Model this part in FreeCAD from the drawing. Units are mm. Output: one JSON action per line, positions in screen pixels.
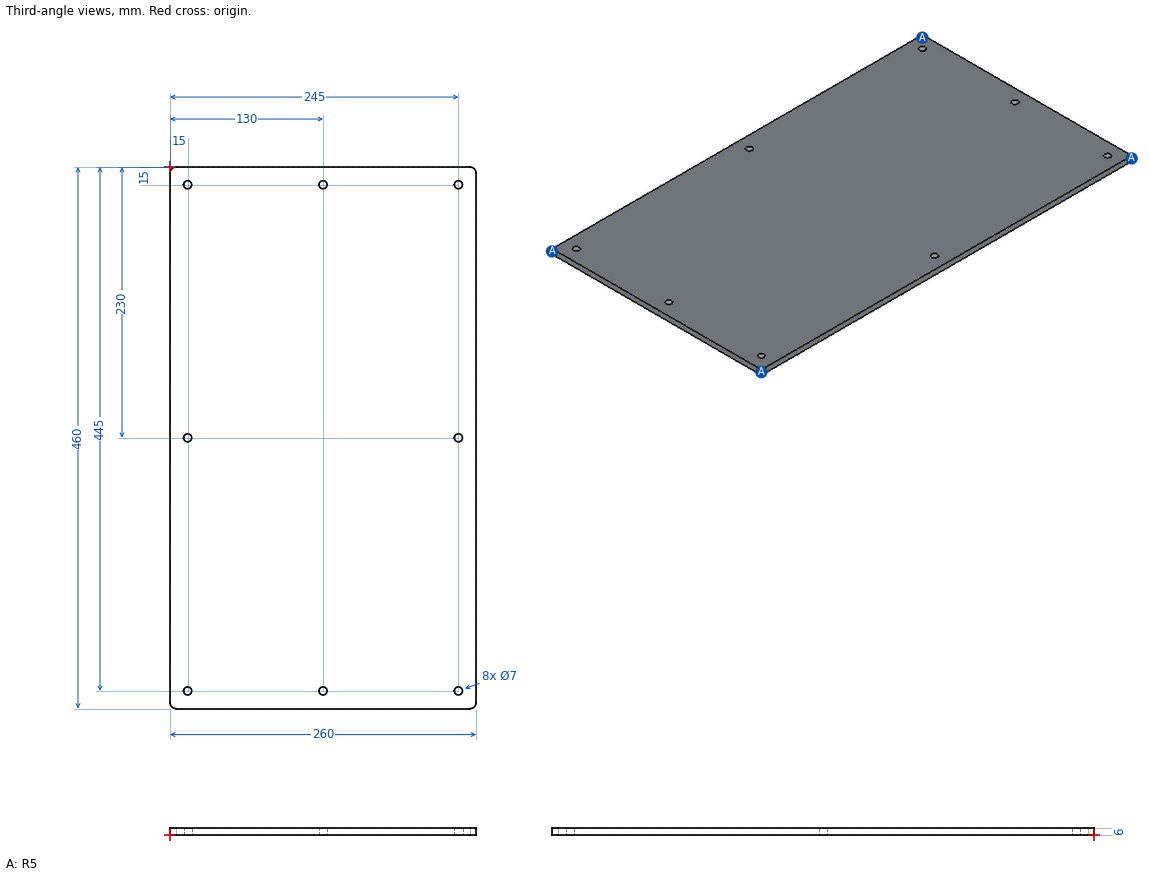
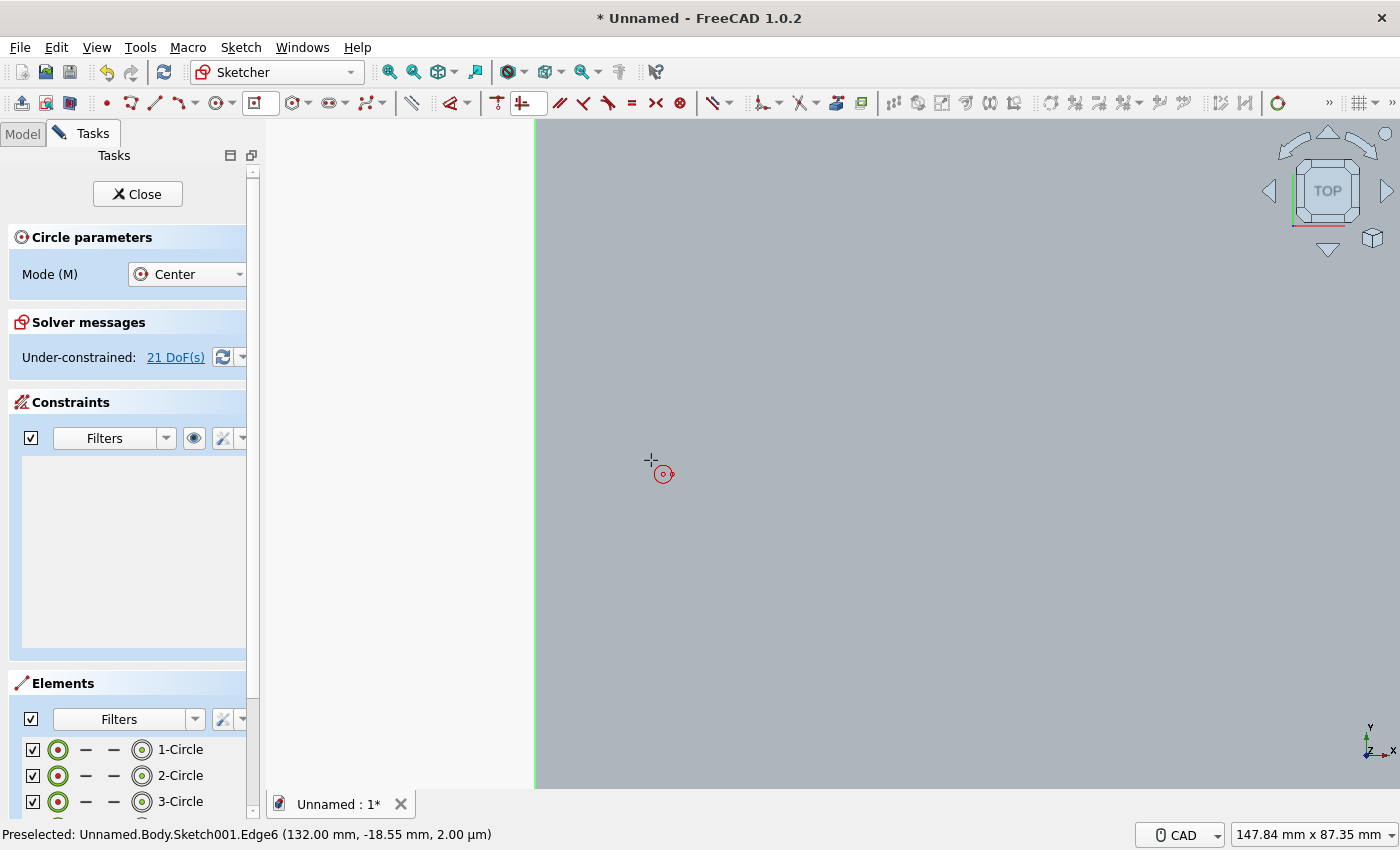
{"action": "scroll", "coordinate": [651, 460], "scroll_direction": "down", "scroll_amount": 10}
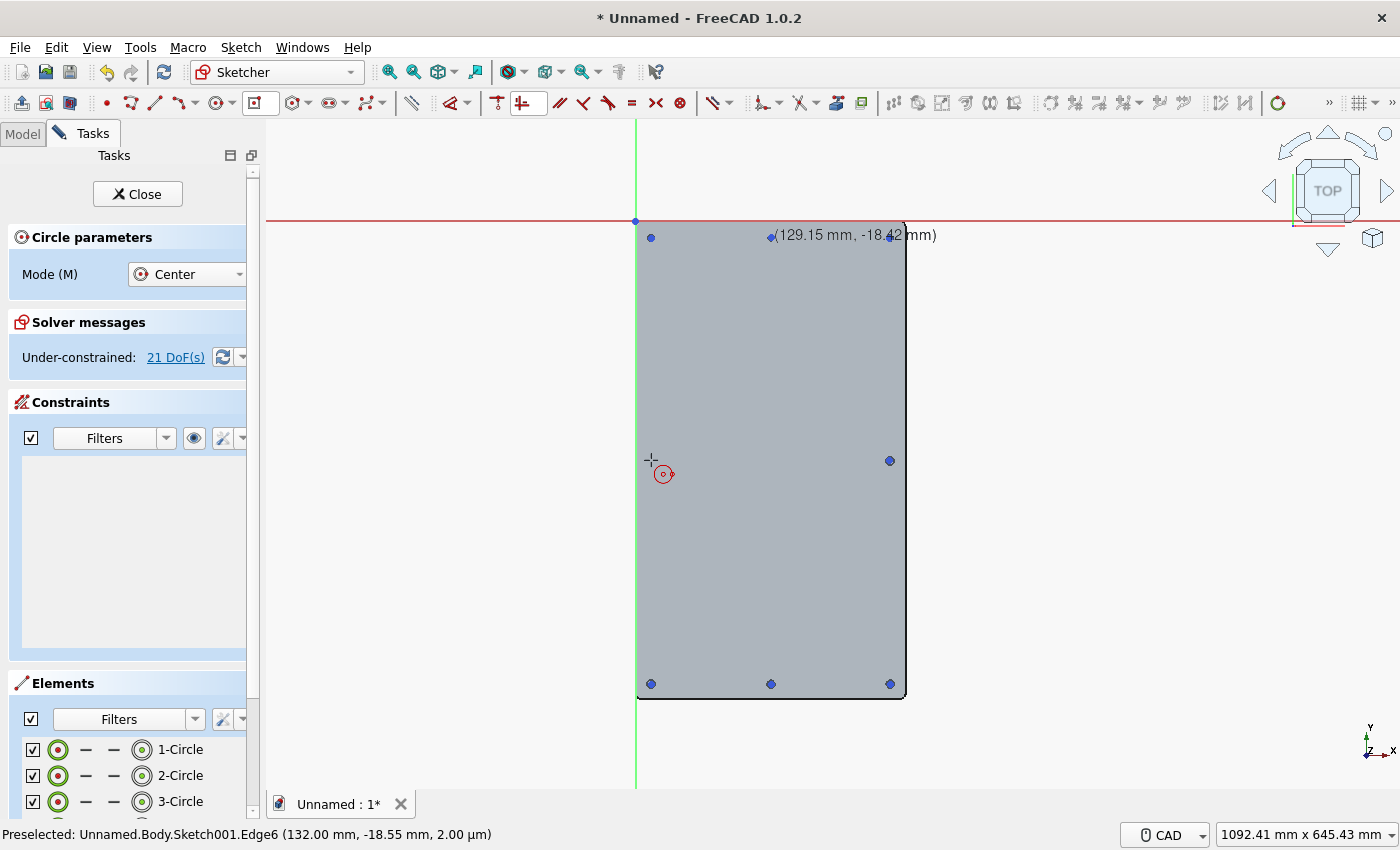
{"action": "left_click", "coordinate": [651, 460]}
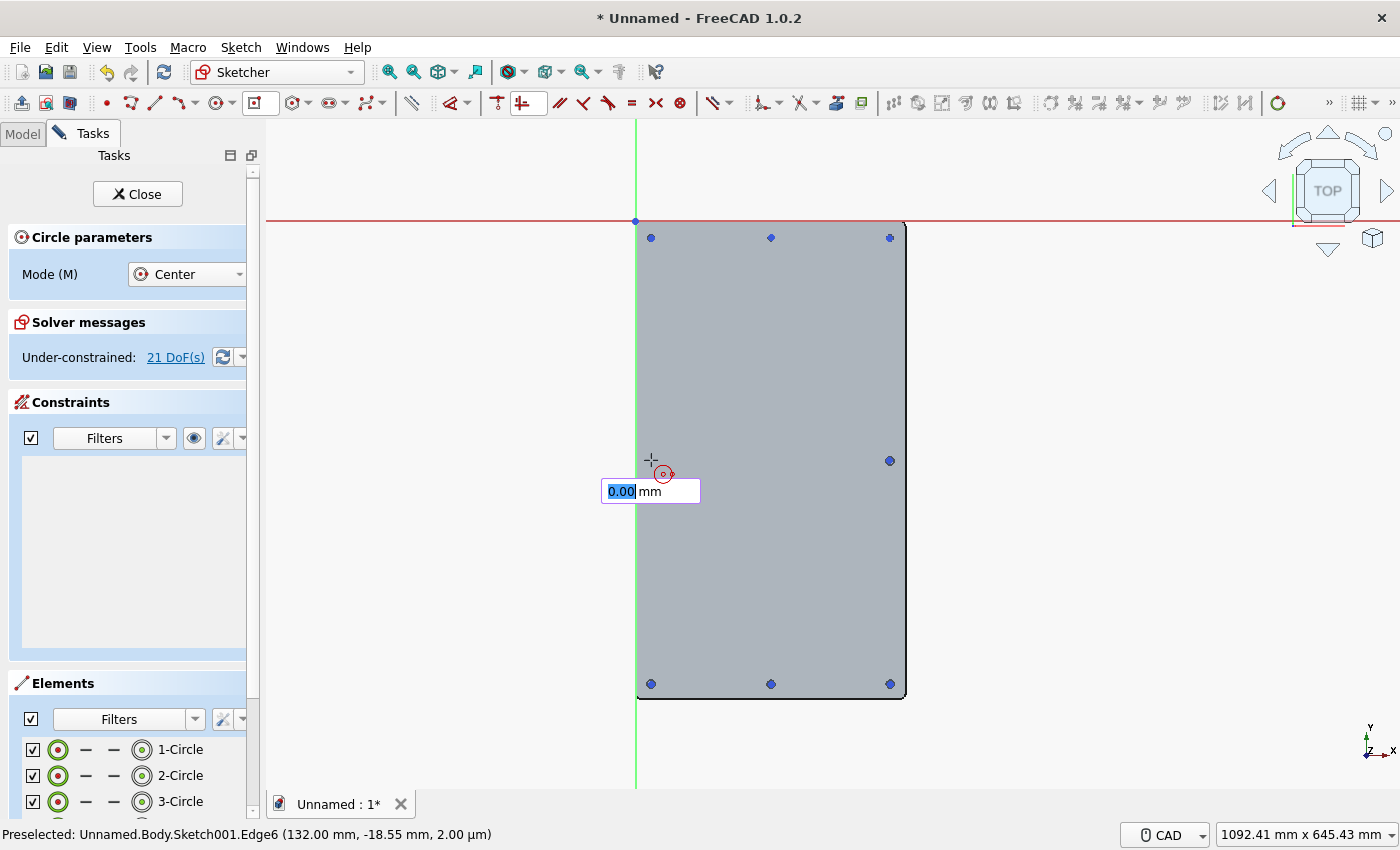
{"action": "scroll", "coordinate": [654, 458], "scroll_direction": "up", "scroll_amount": 8}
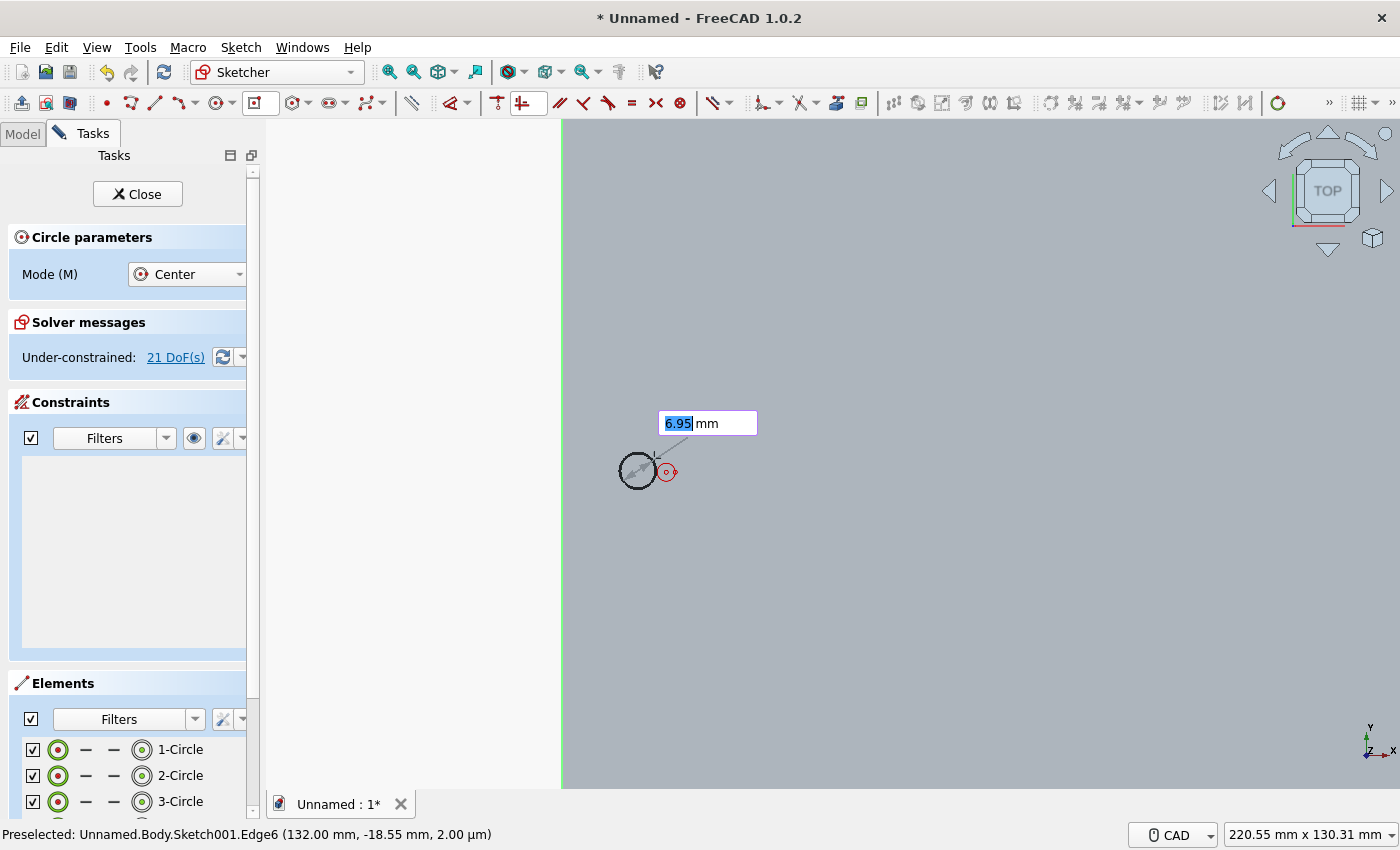
{"action": "left_click", "coordinate": [651, 454]}
{"action": "key", "text": "Escape"}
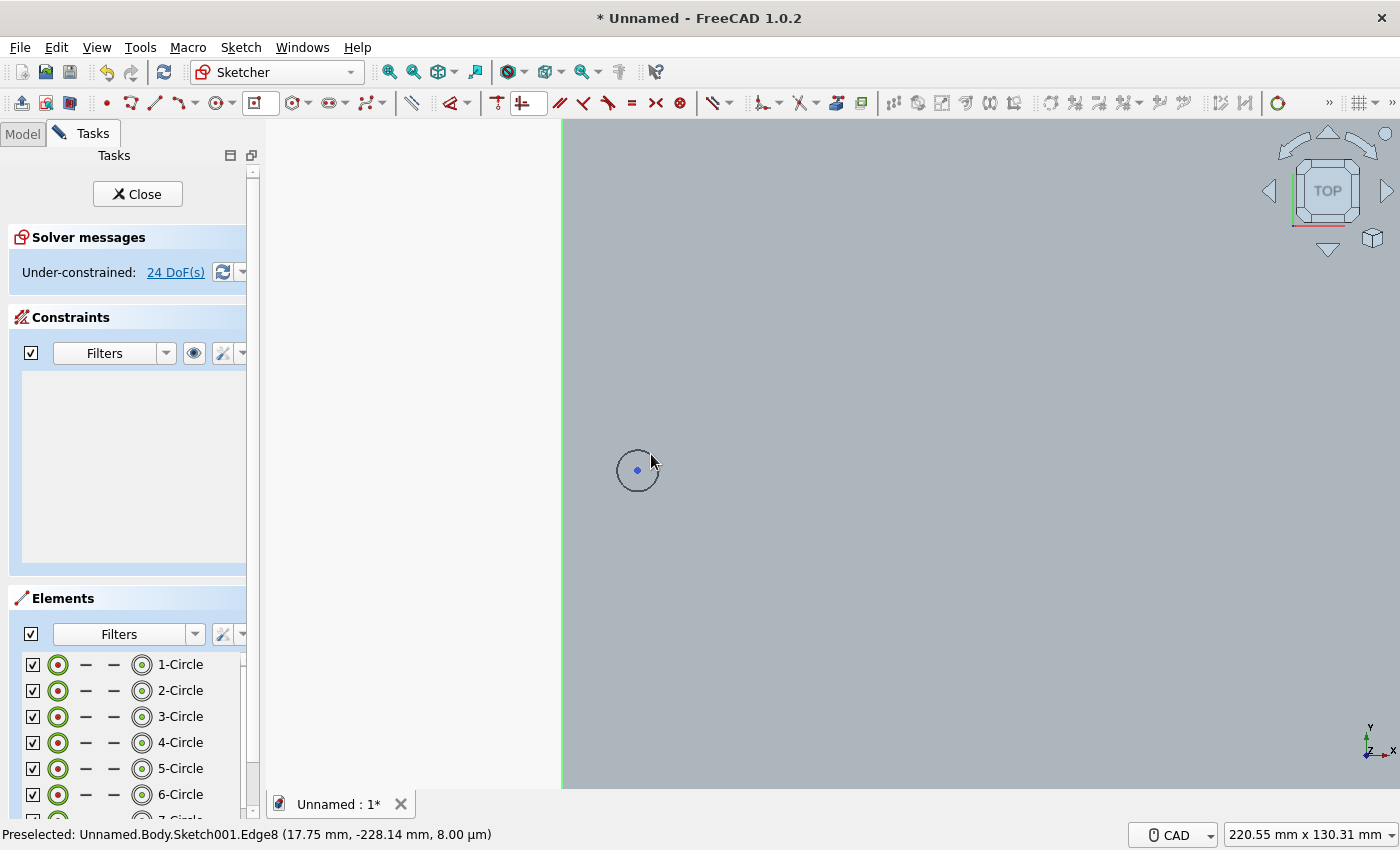
{"action": "scroll", "coordinate": [654, 458], "scroll_direction": "down", "scroll_amount": 8}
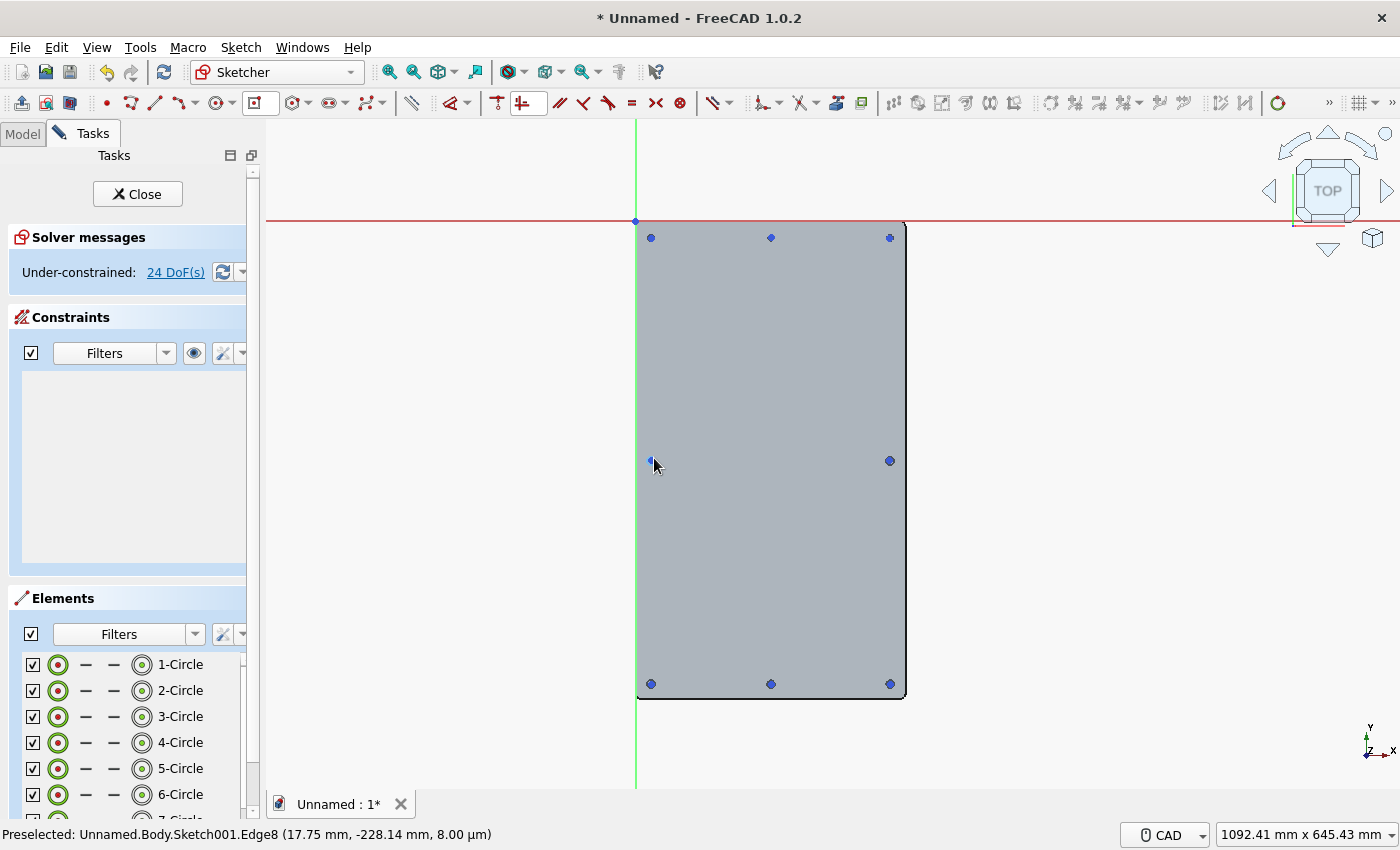
{"action": "scroll", "coordinate": [893, 681], "scroll_direction": "up", "scroll_amount": 7}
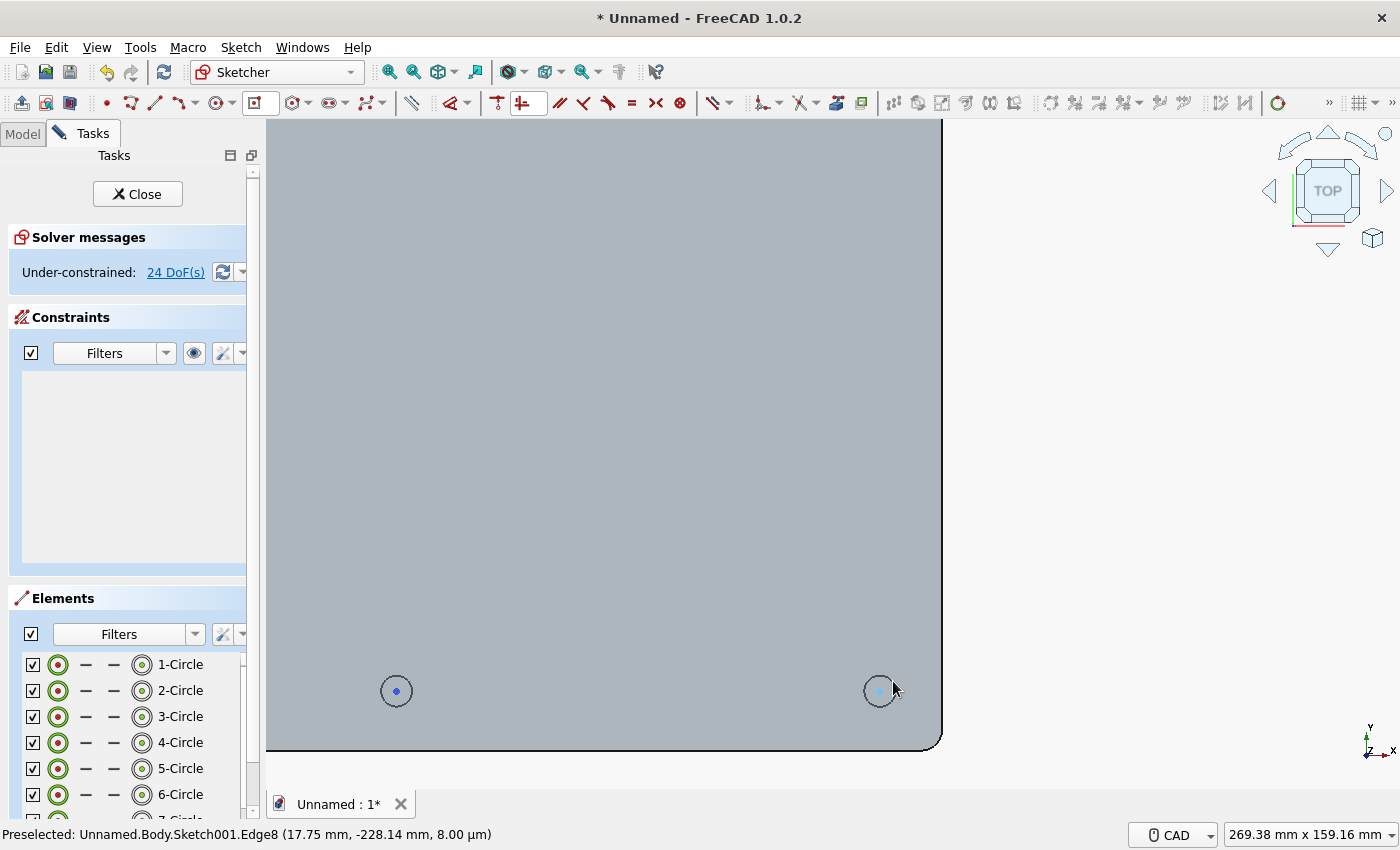
{"action": "left_click", "coordinate": [891, 680]}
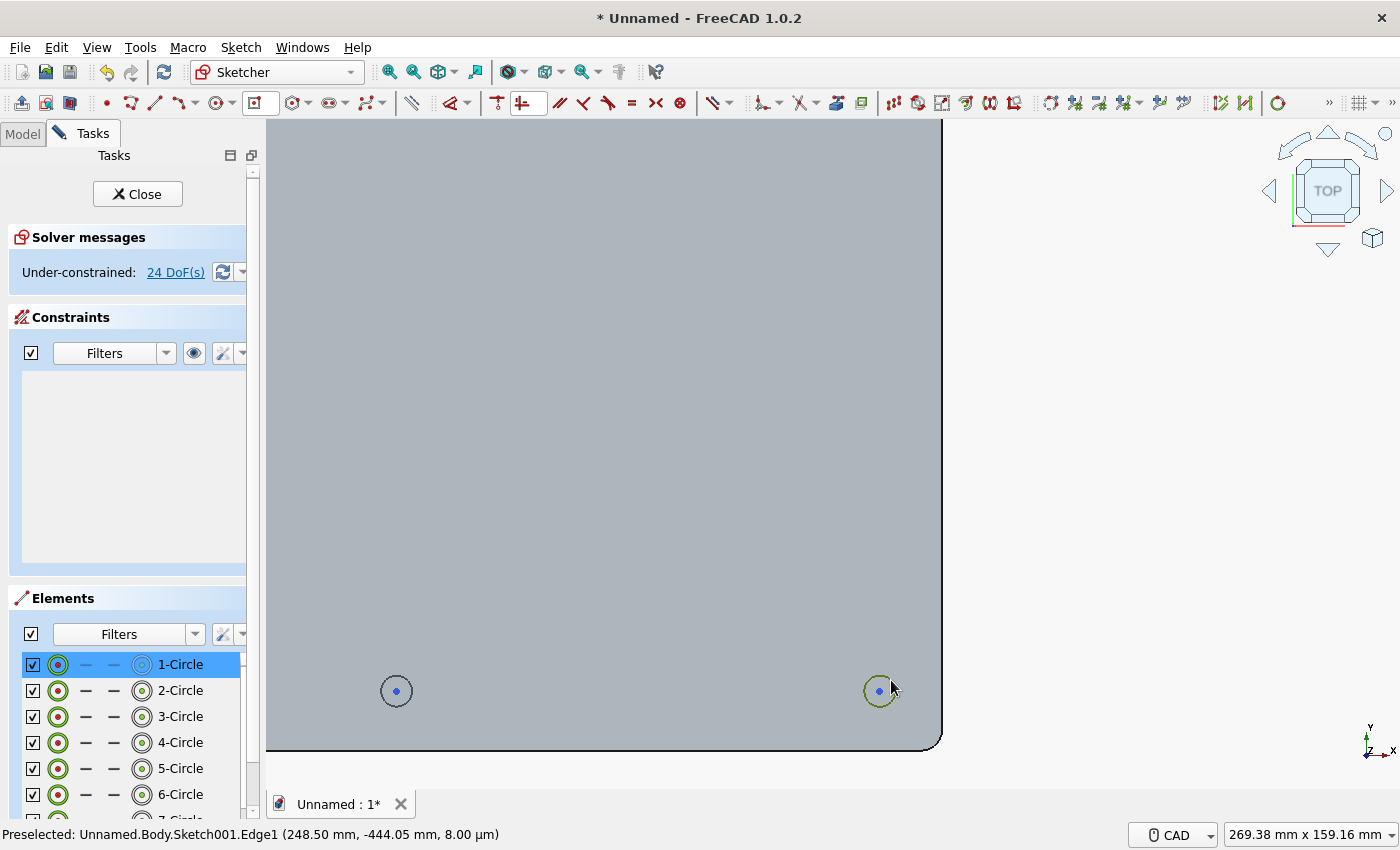
{"action": "scroll", "coordinate": [893, 682], "scroll_direction": "down", "scroll_amount": 7}